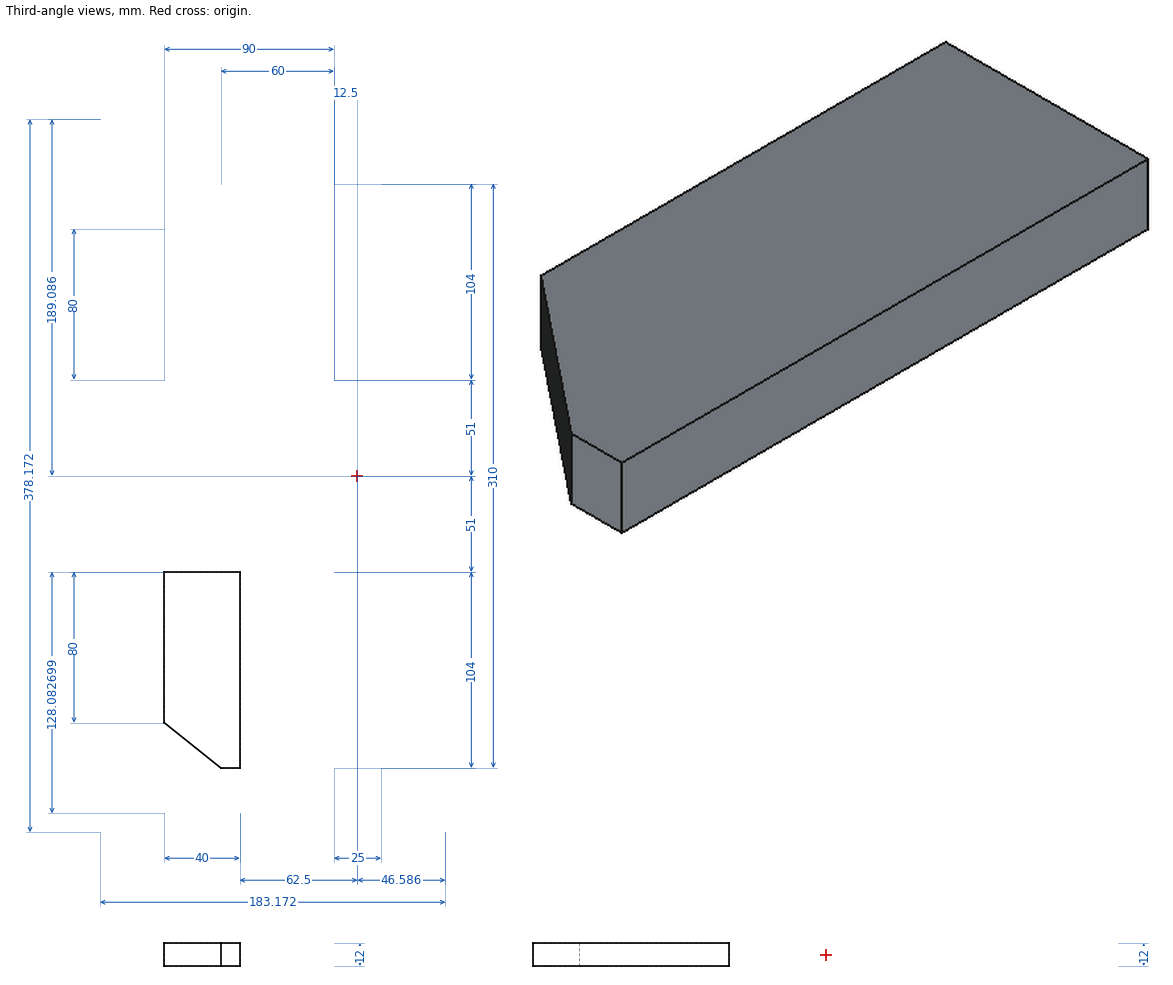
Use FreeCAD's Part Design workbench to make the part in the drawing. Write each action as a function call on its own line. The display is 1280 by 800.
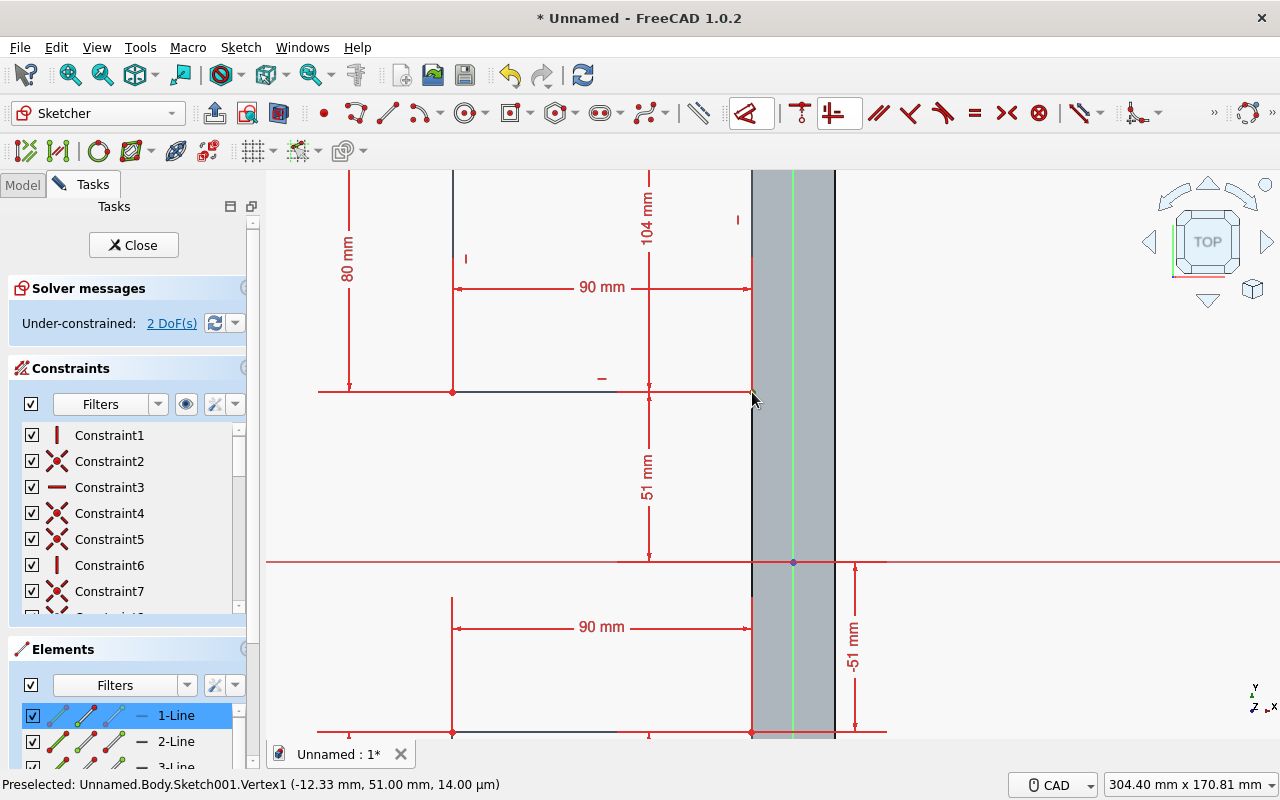
click(768, 114)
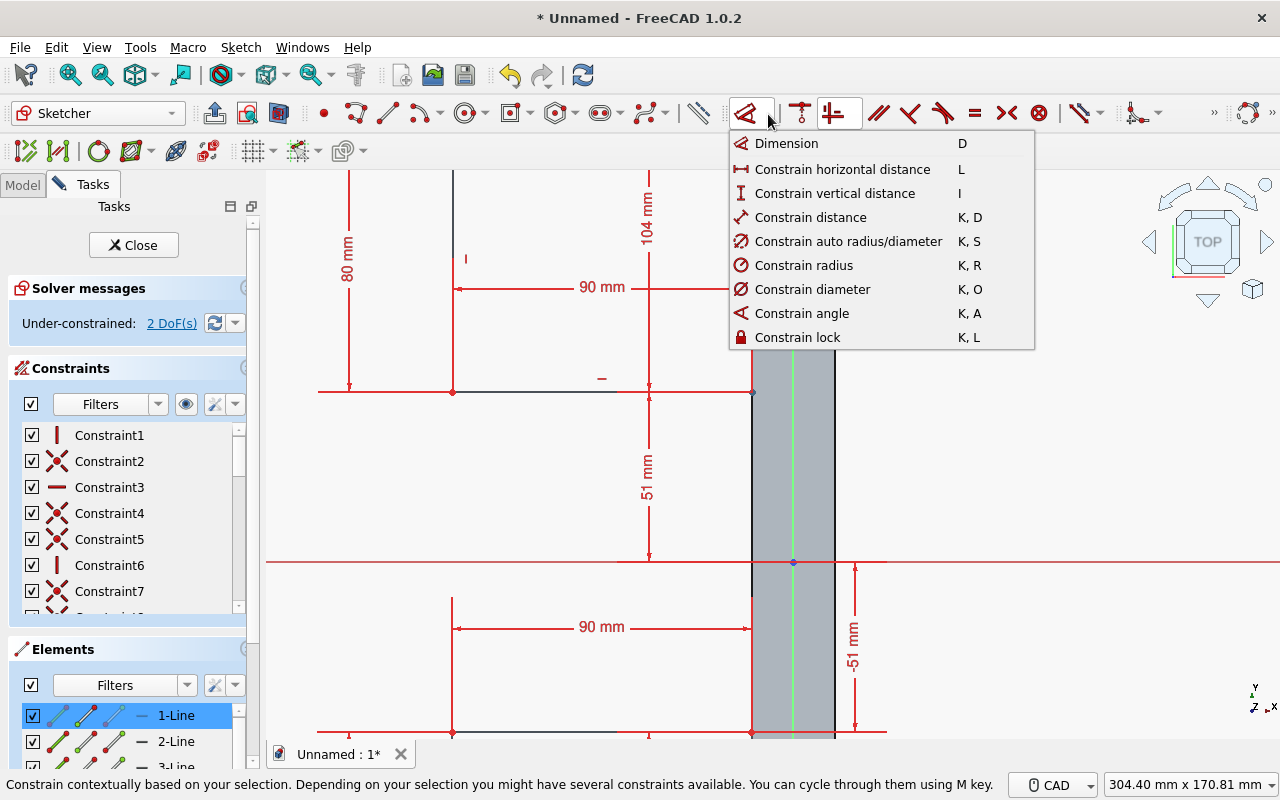
click(882, 169)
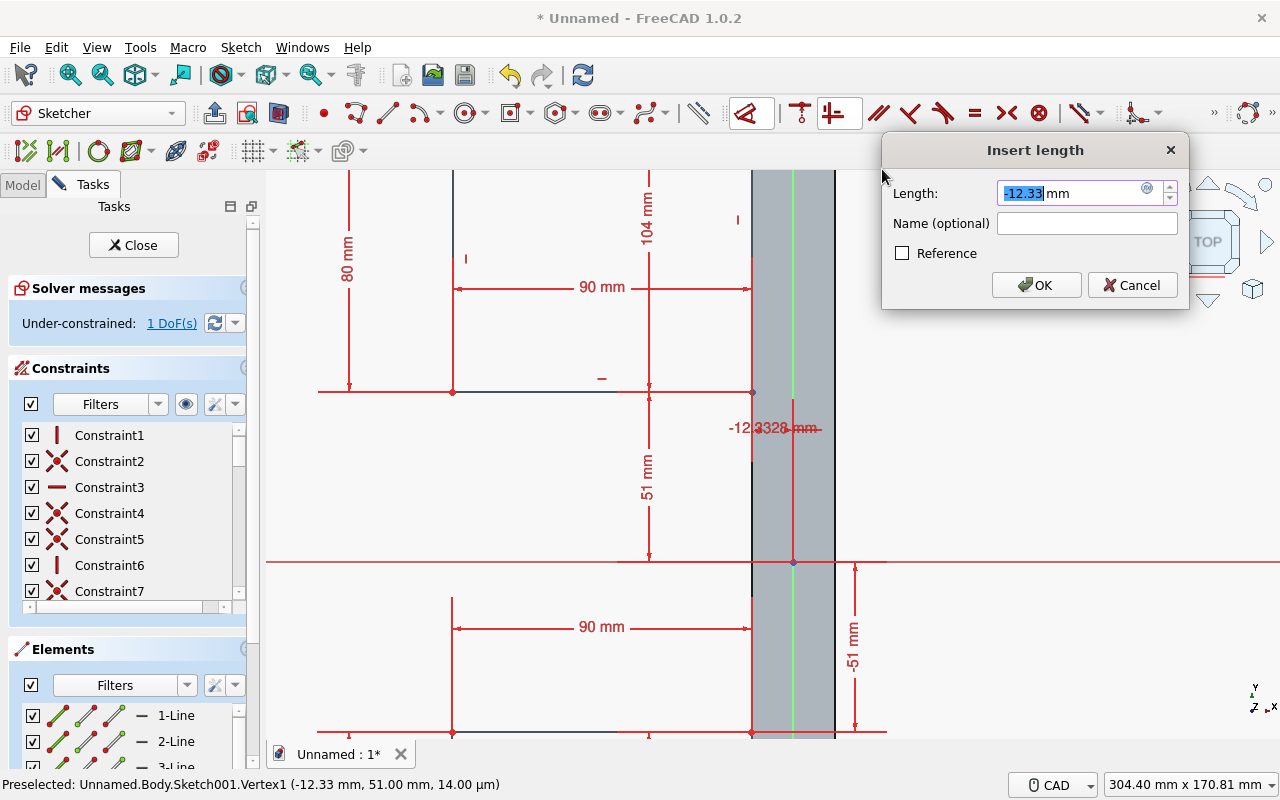
text(-12.5)
key(Return)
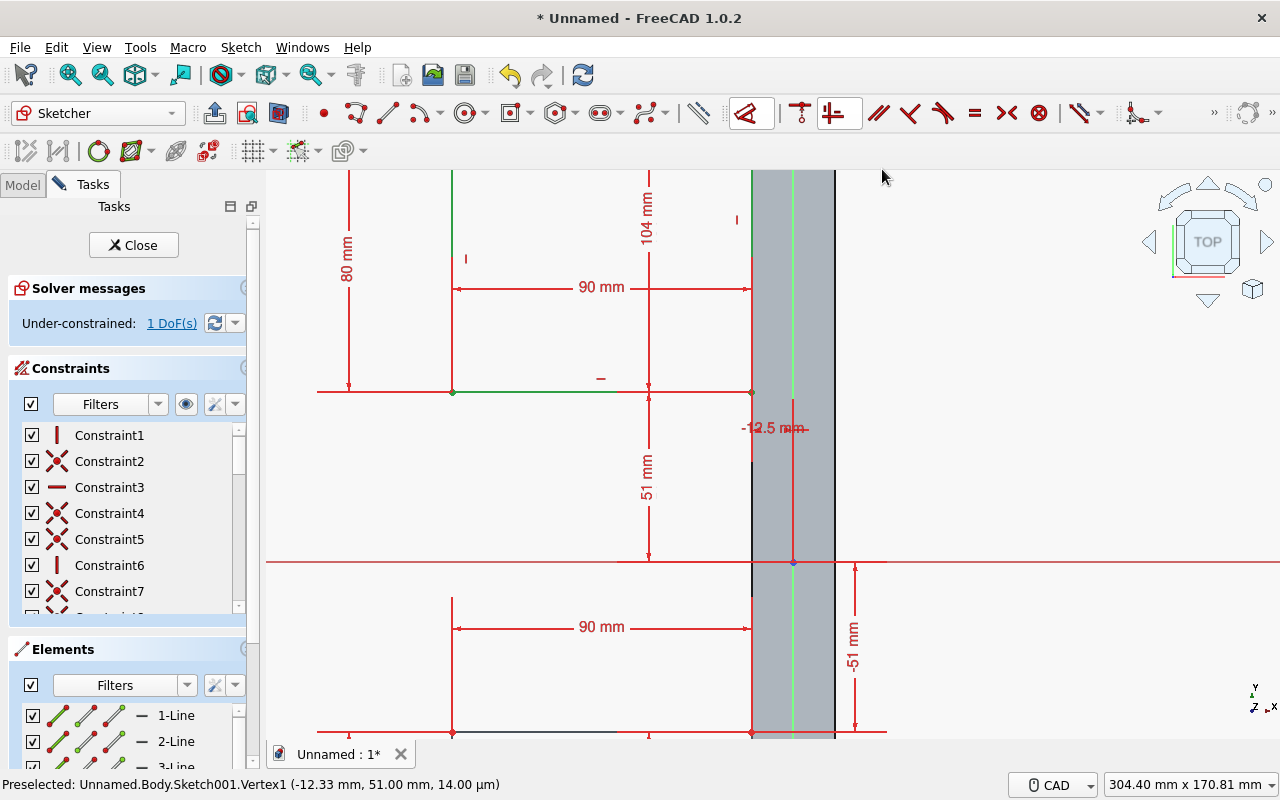
scroll(752, 392, down, 5)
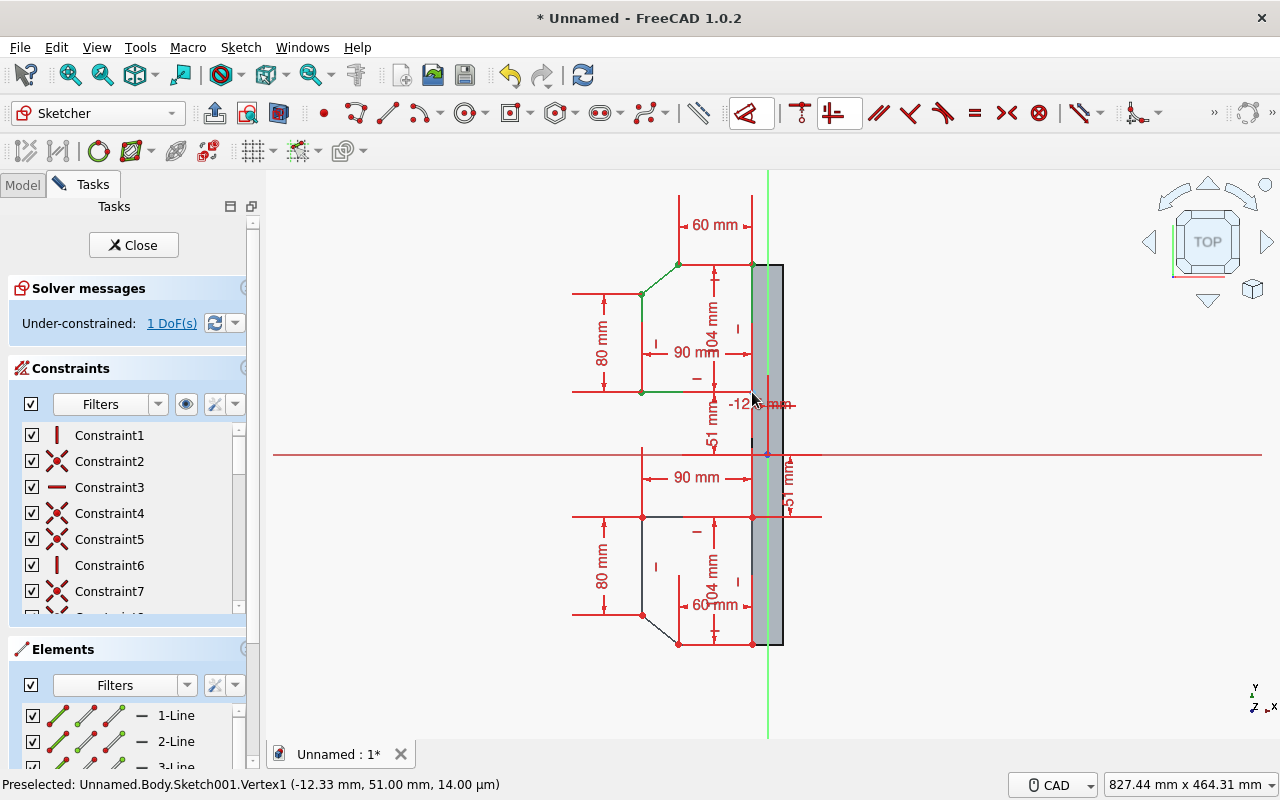
scroll(752, 517, up, 5)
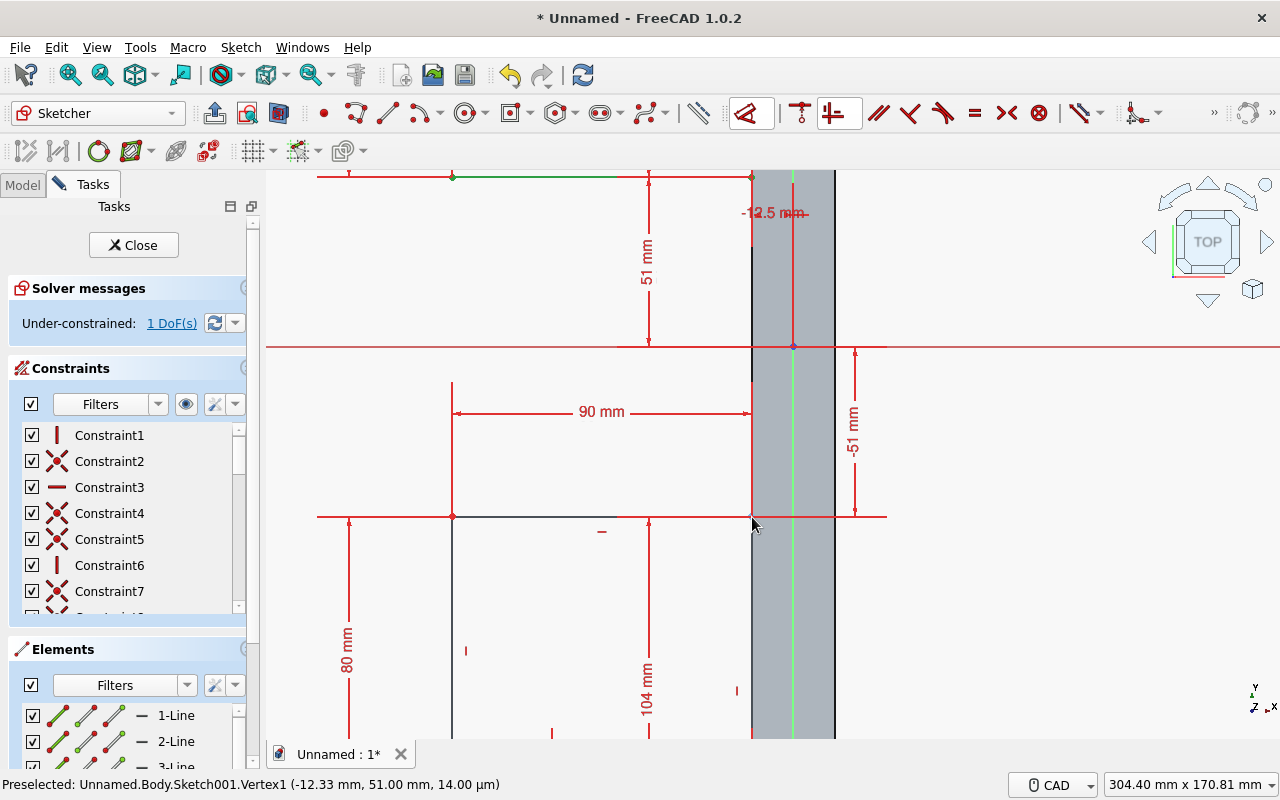
click(752, 517)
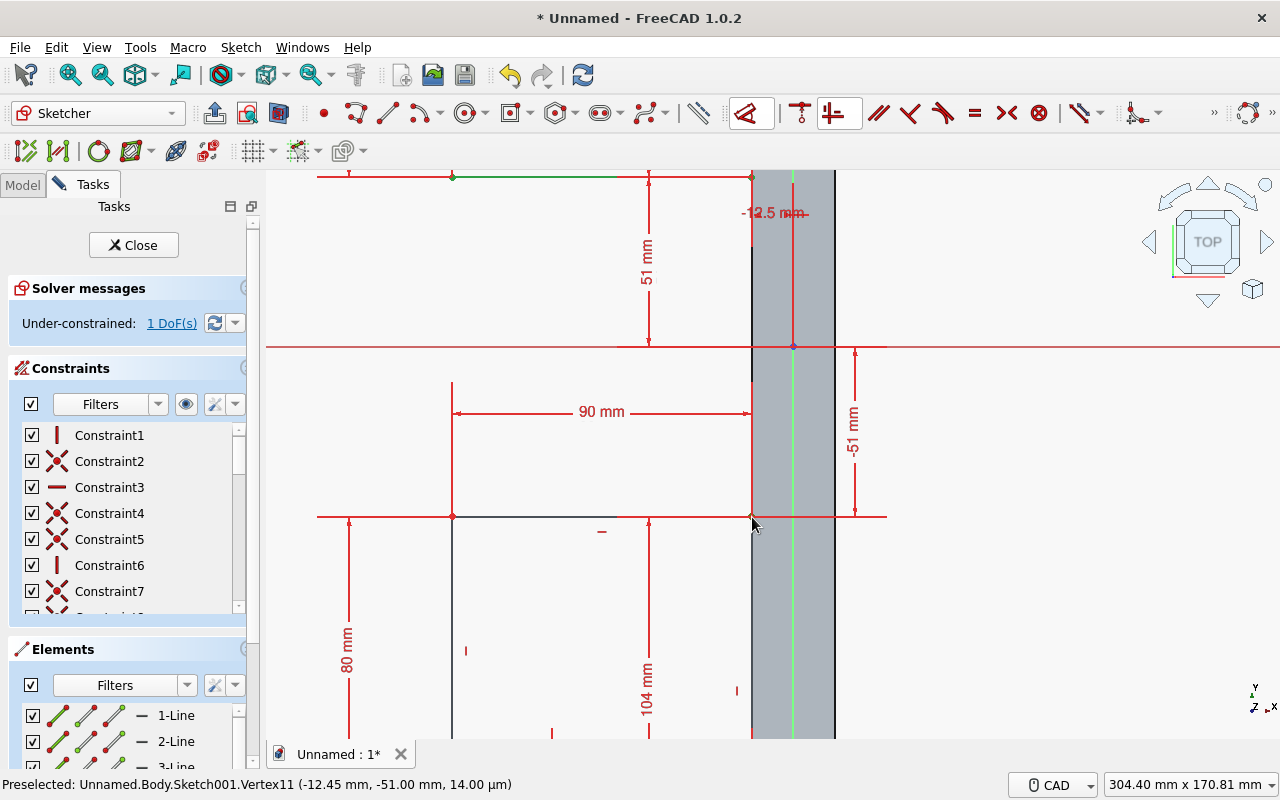
click(768, 114)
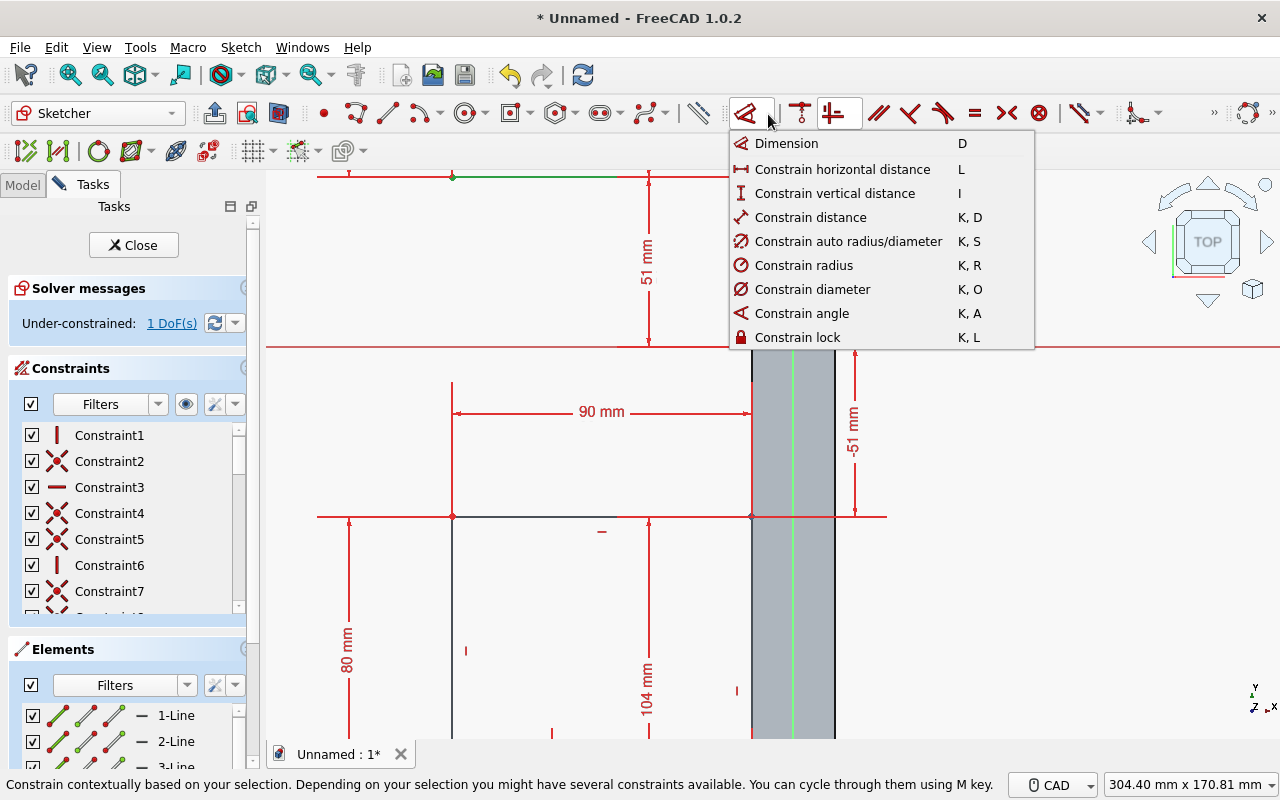
click(882, 169)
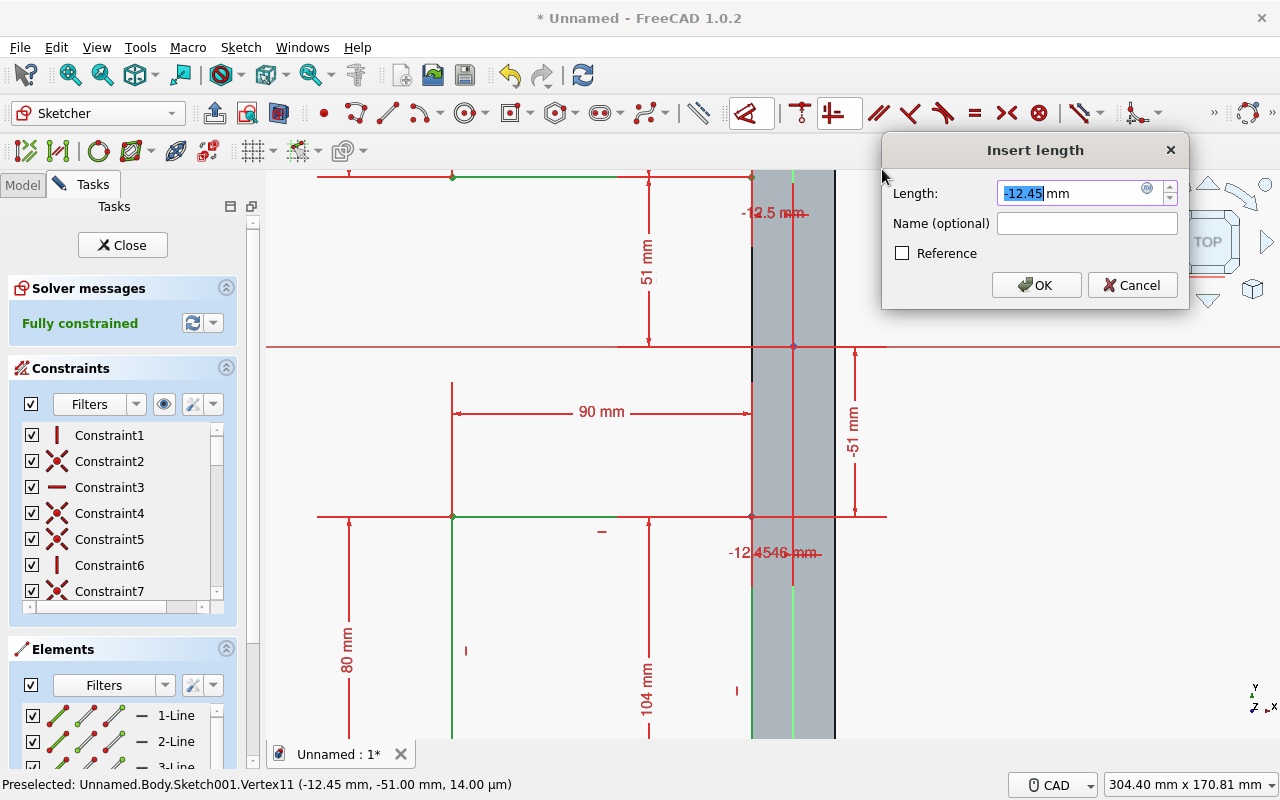
text(-12.5)
key(Return)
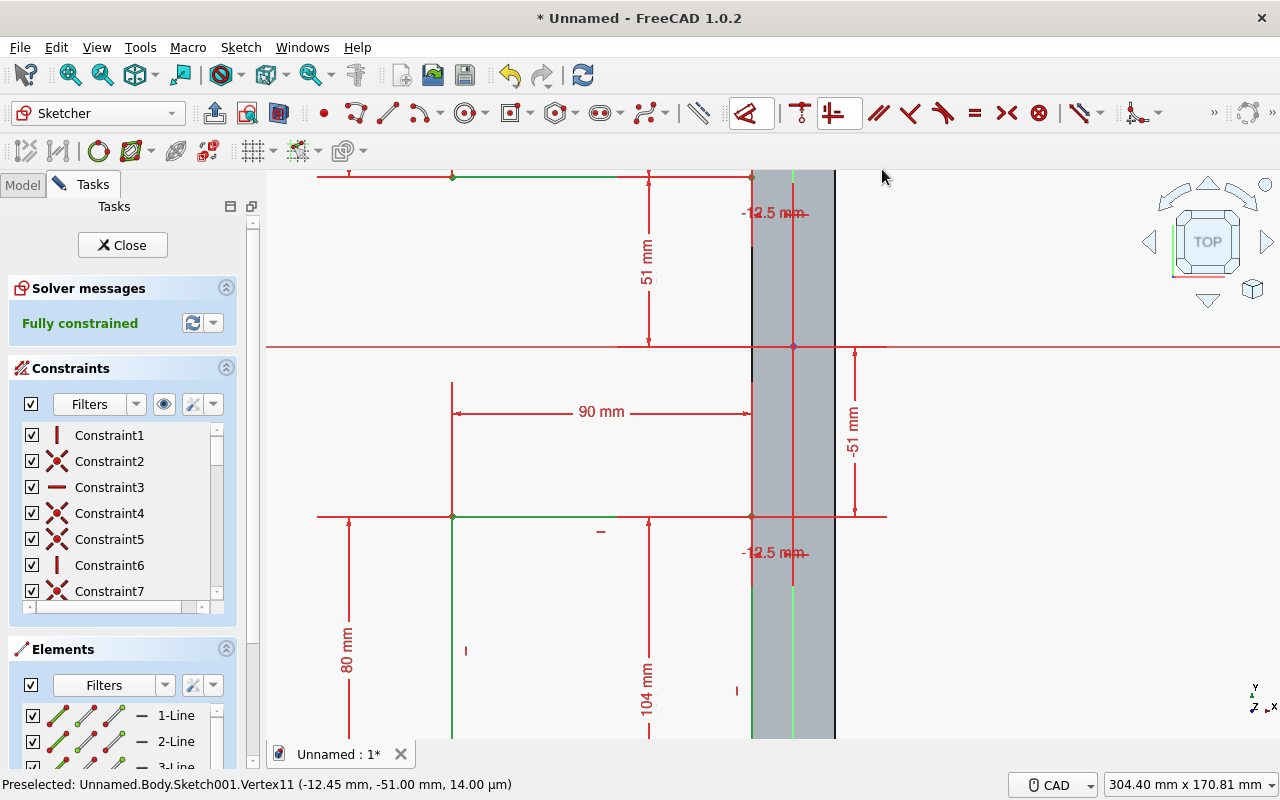
click(123, 245)